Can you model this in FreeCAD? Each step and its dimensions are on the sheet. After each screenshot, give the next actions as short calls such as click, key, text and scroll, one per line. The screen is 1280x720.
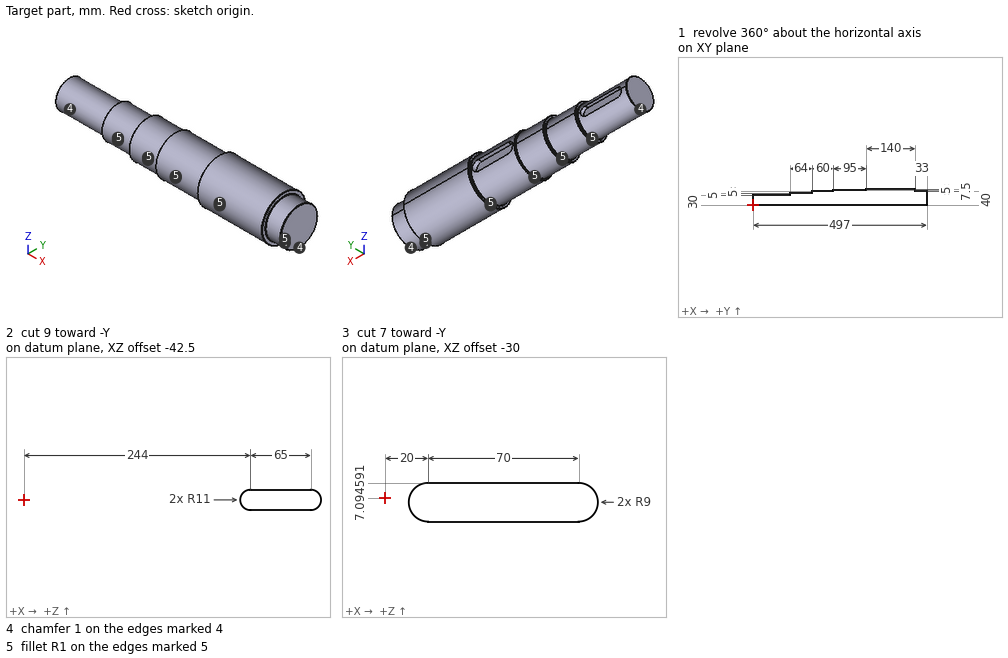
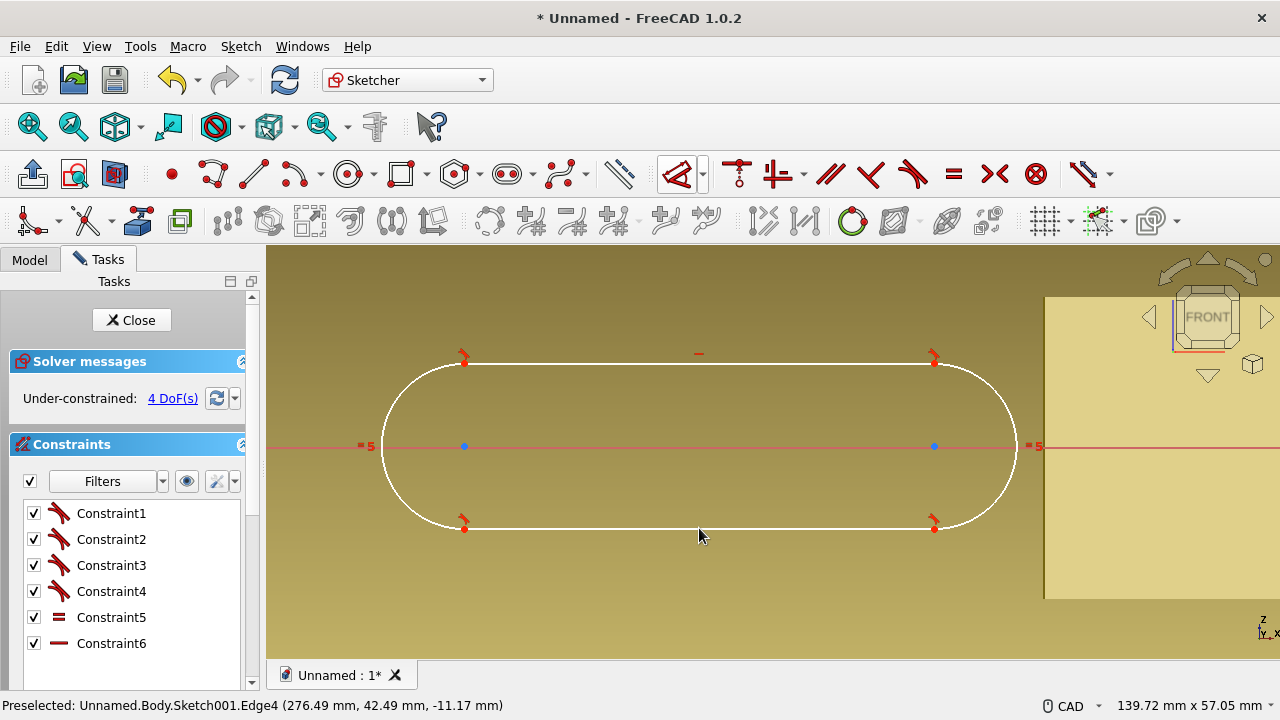
click(464, 446)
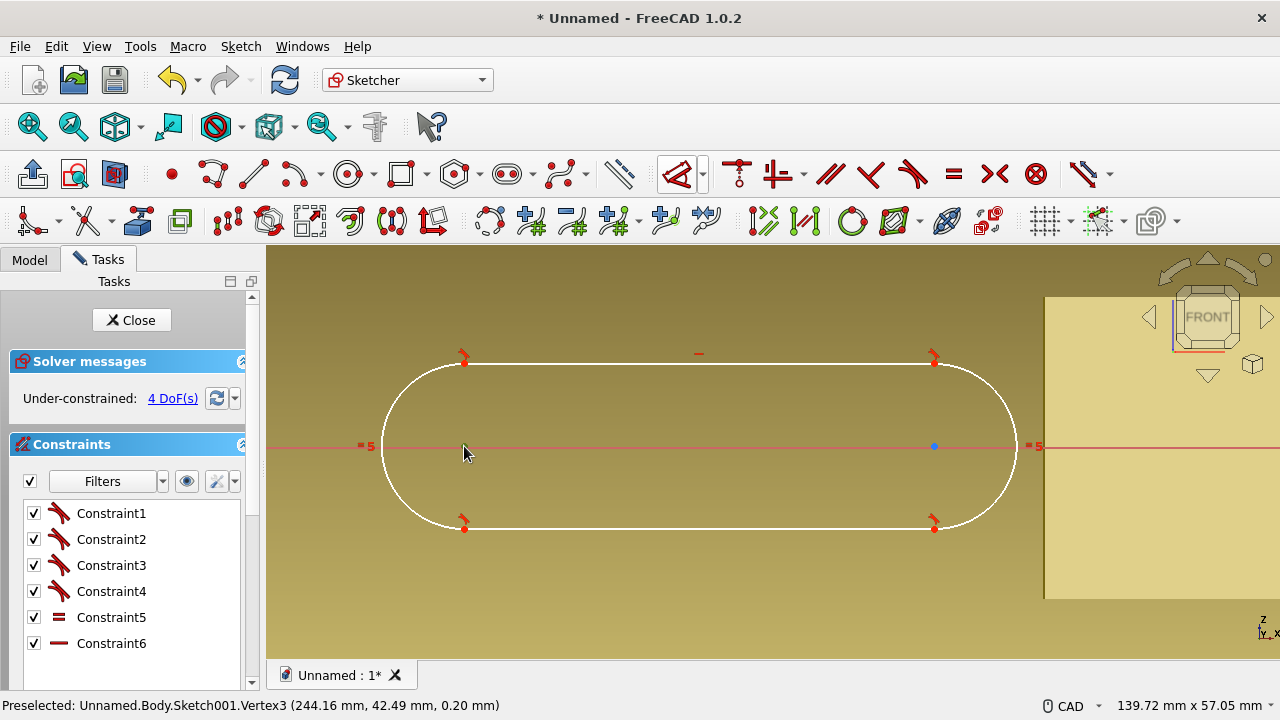
click(470, 448)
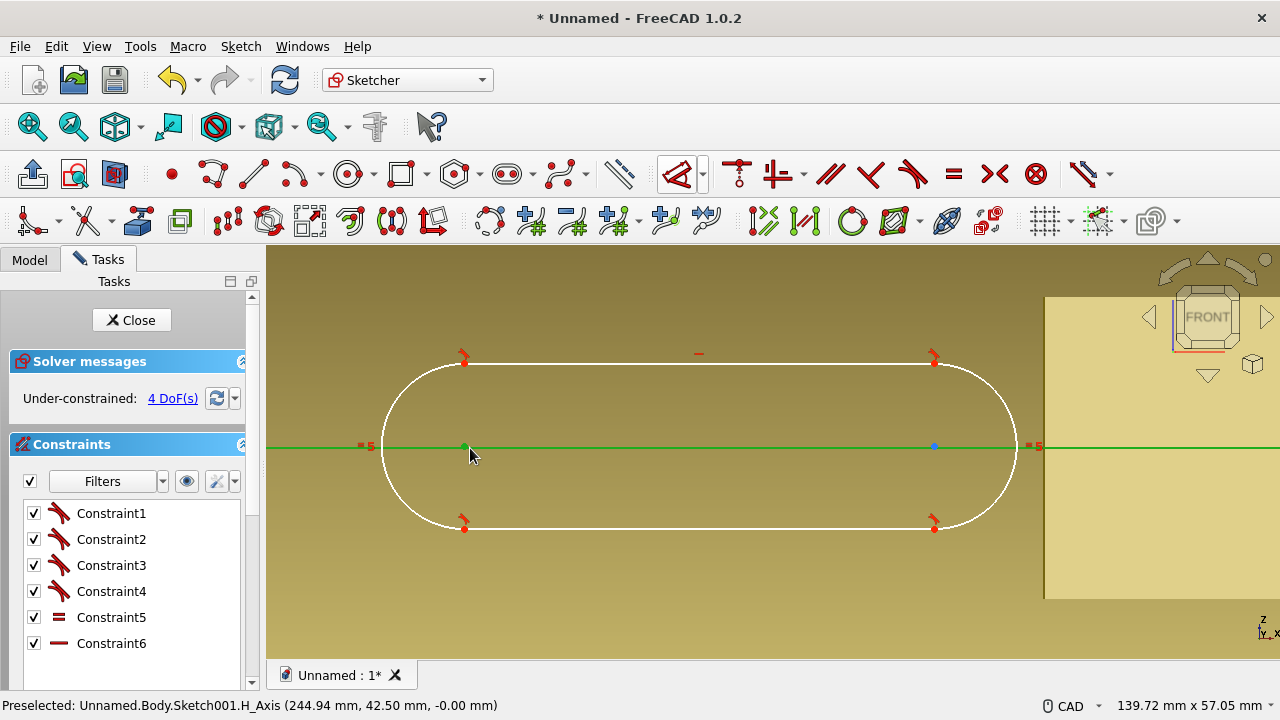
click(737, 174)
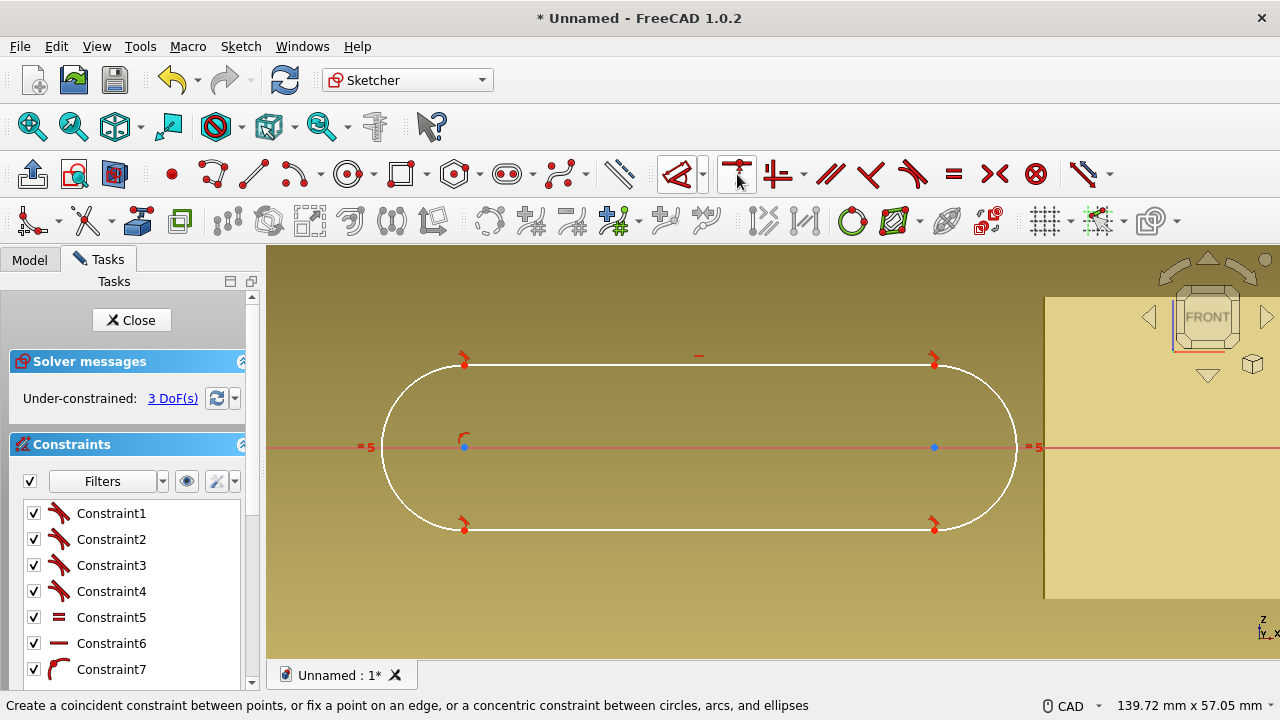
click(398, 399)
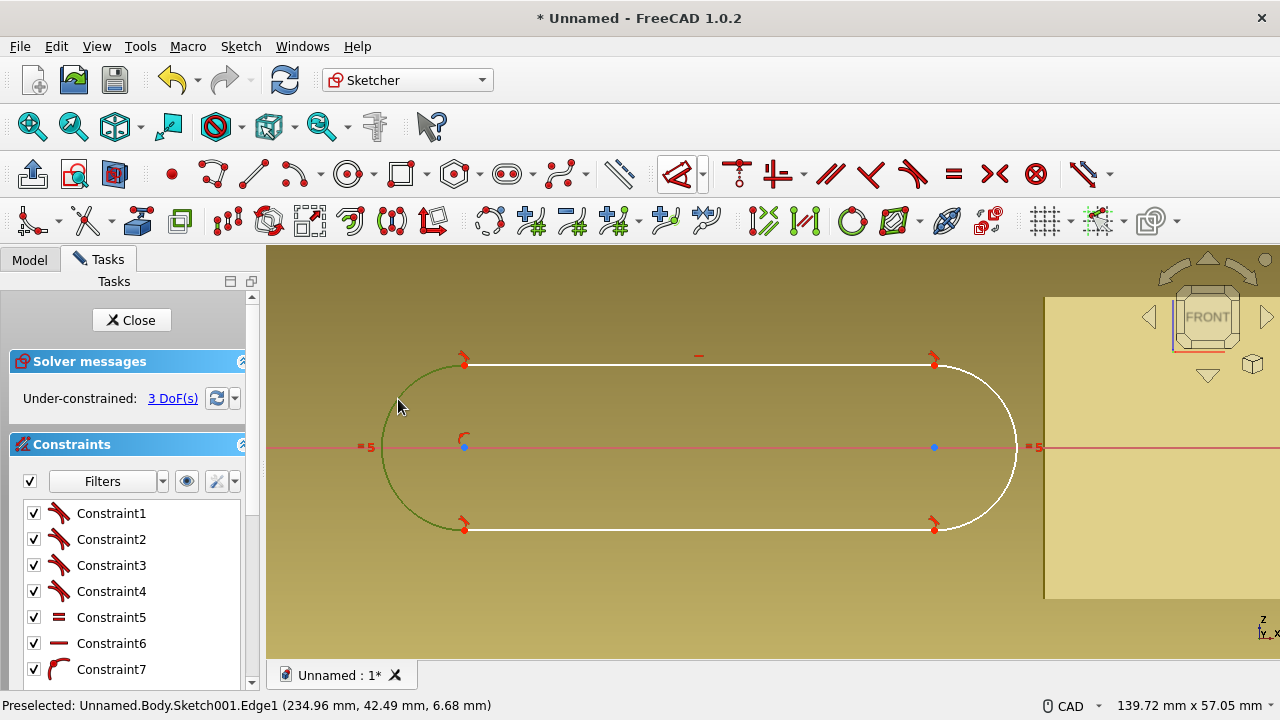
key(k)
key(r)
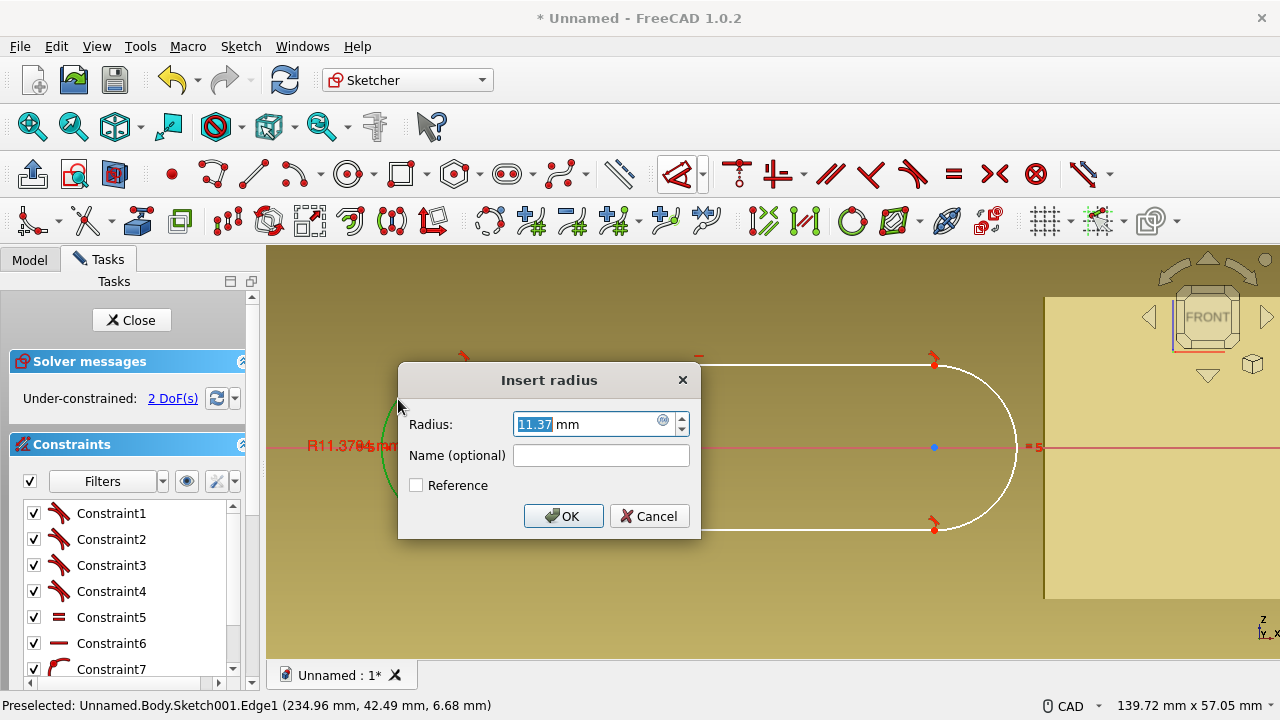
text(11)
key(Return)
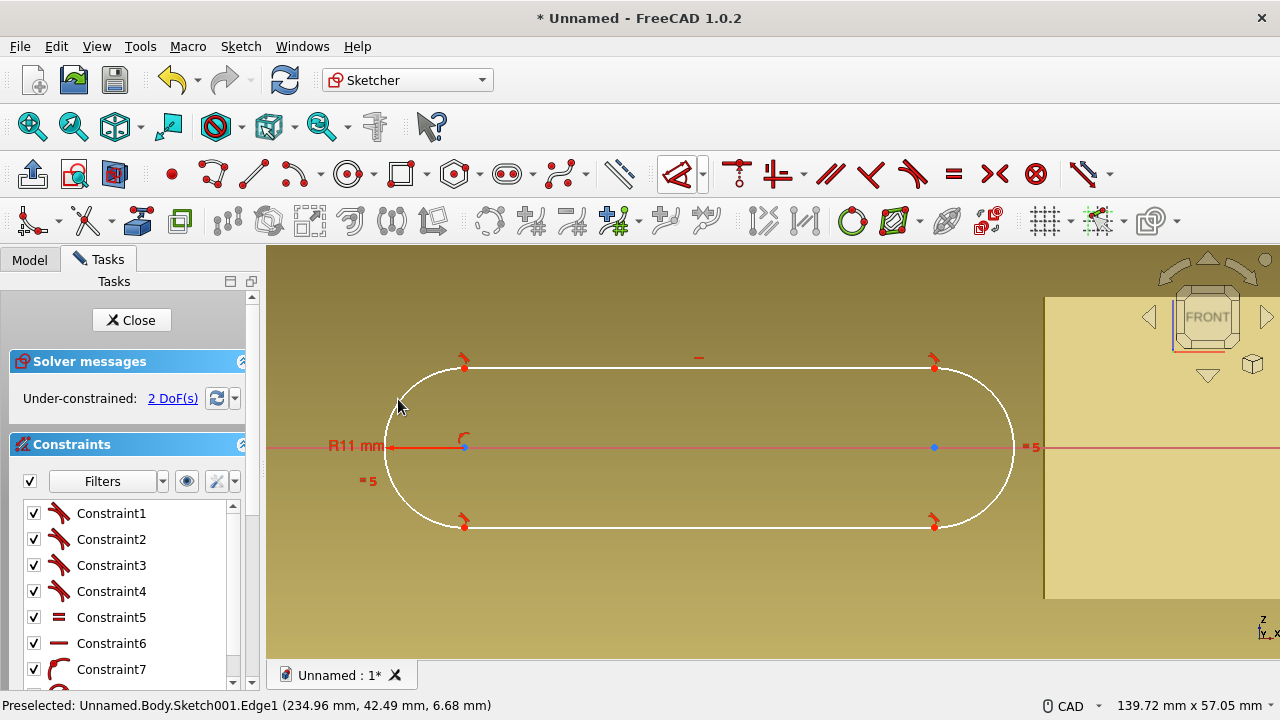
click(605, 368)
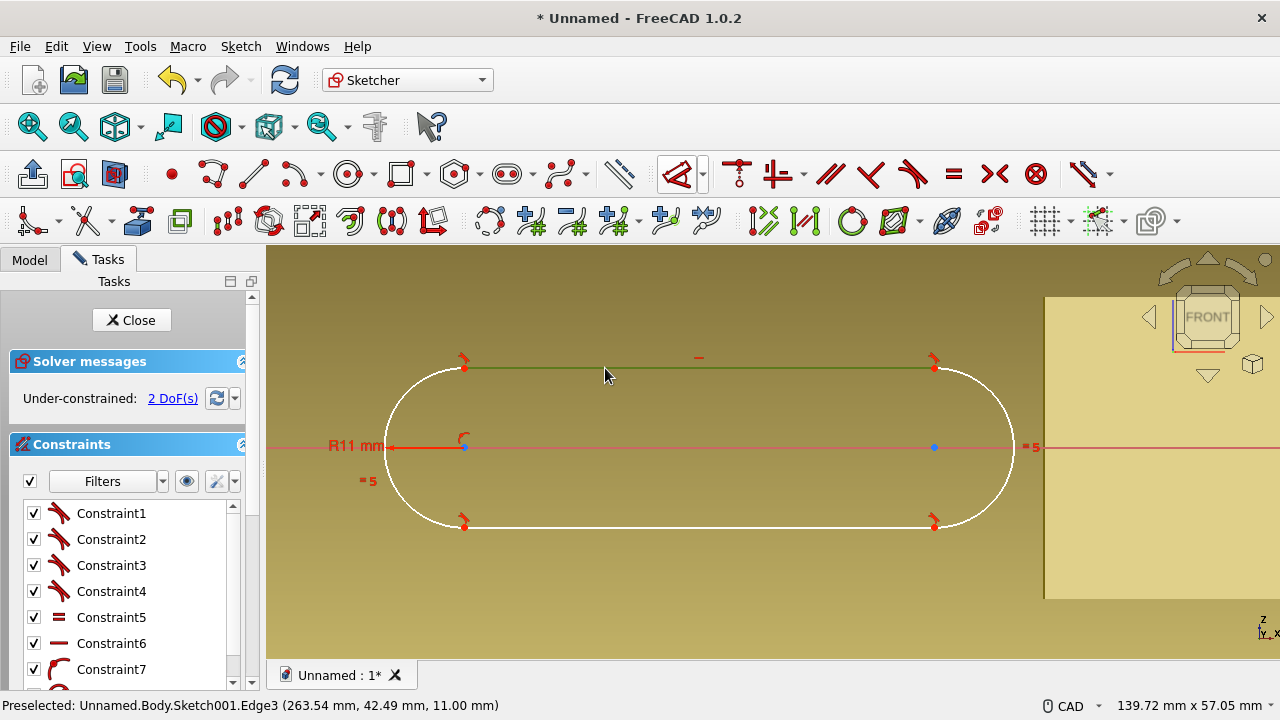
click(702, 174)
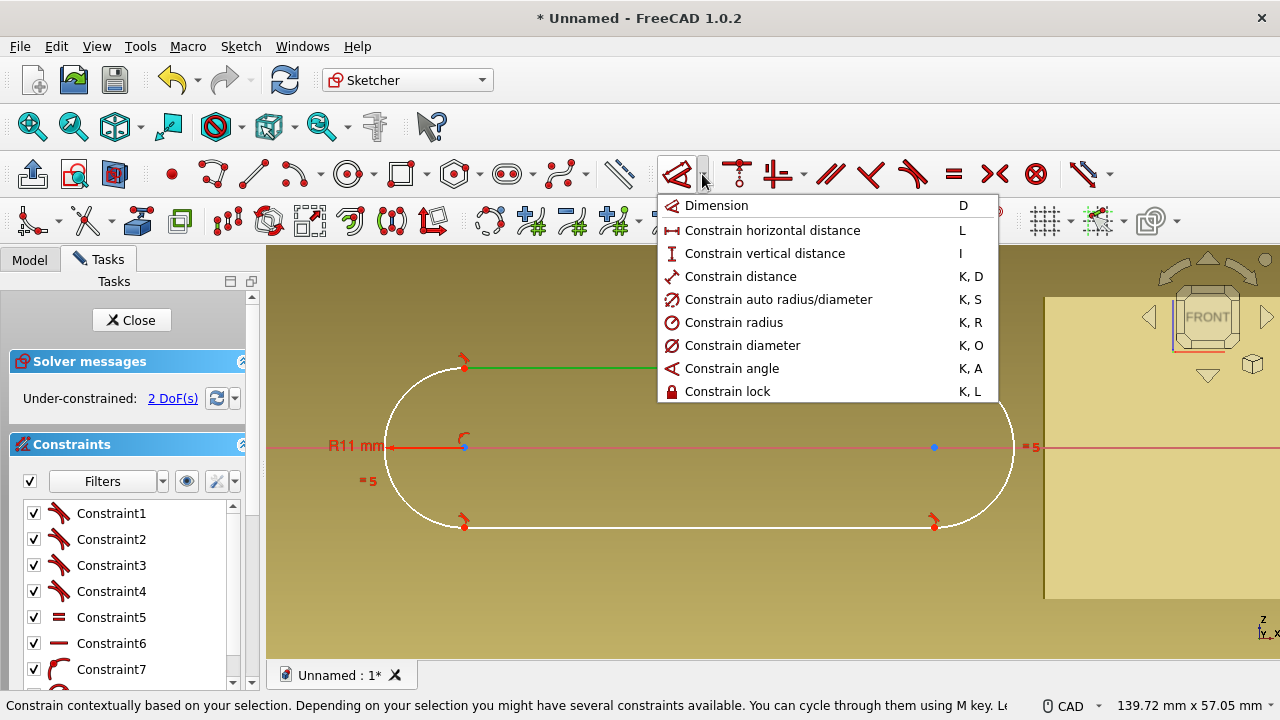
click(828, 230)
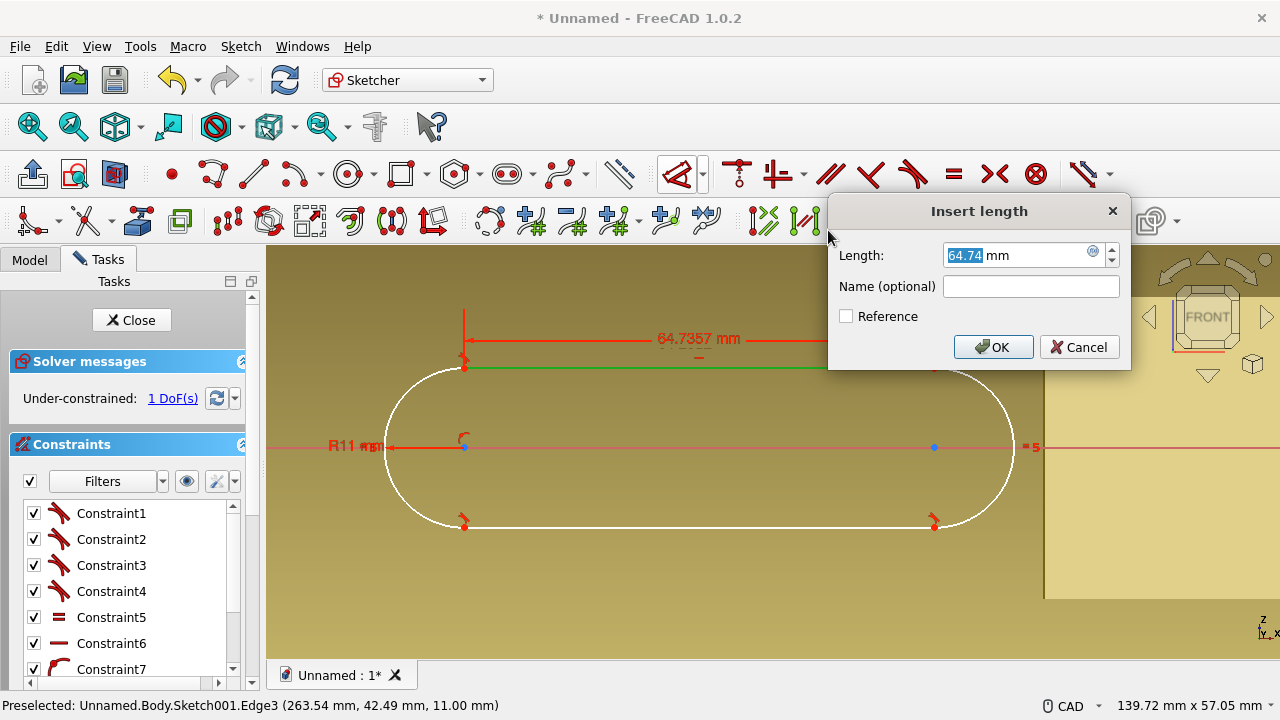
text(65)
key(Return)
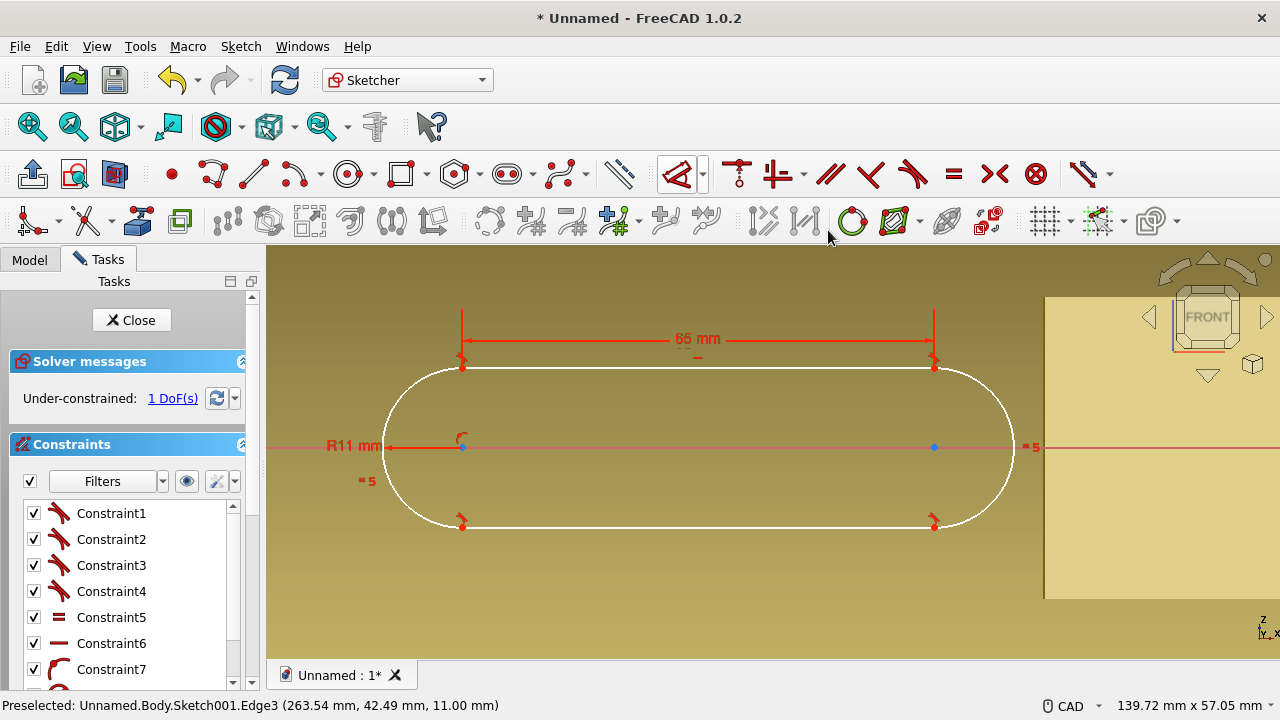
click(462, 368)